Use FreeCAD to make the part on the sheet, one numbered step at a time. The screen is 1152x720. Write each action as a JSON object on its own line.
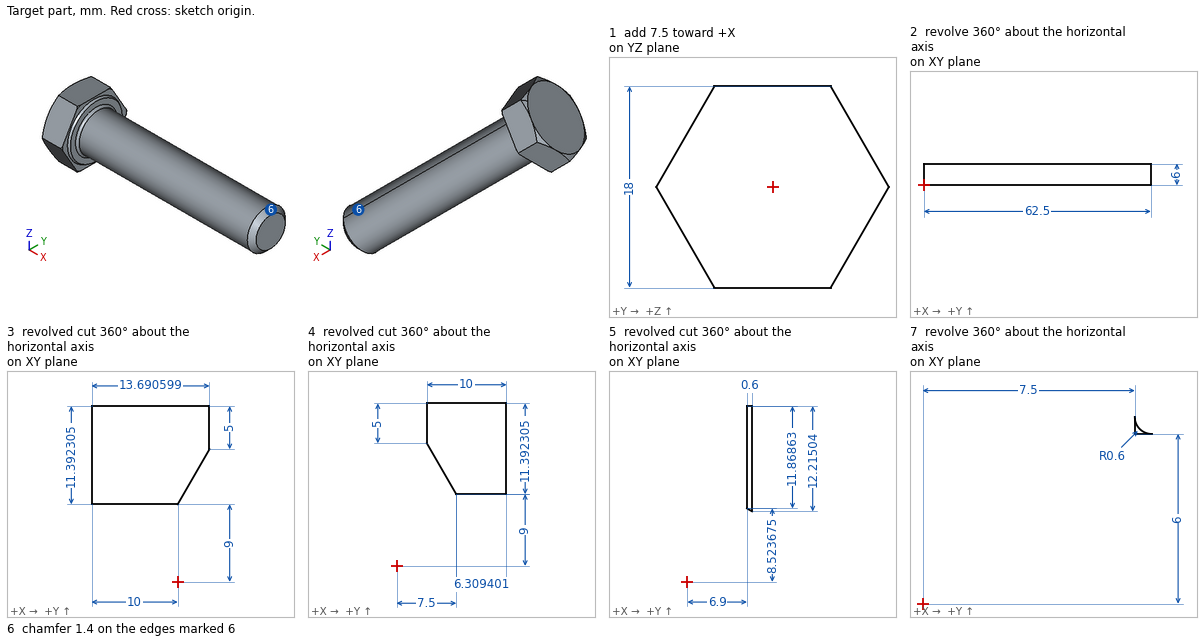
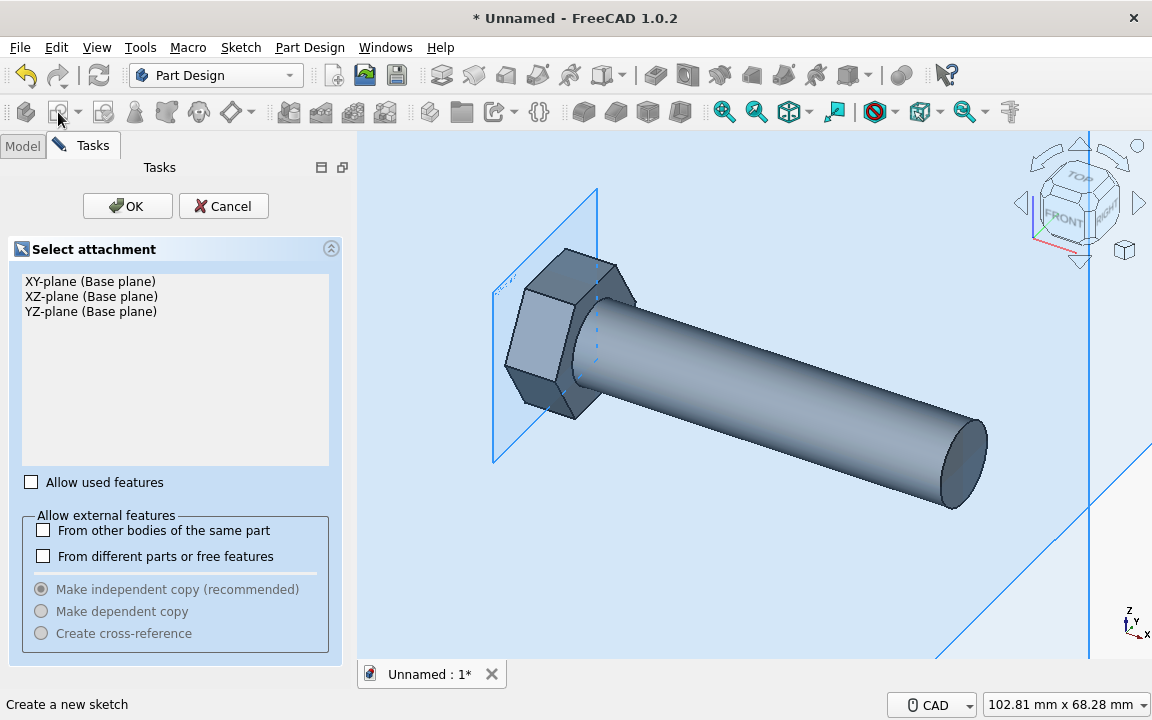
{"action": "left_click", "coordinate": [82, 282]}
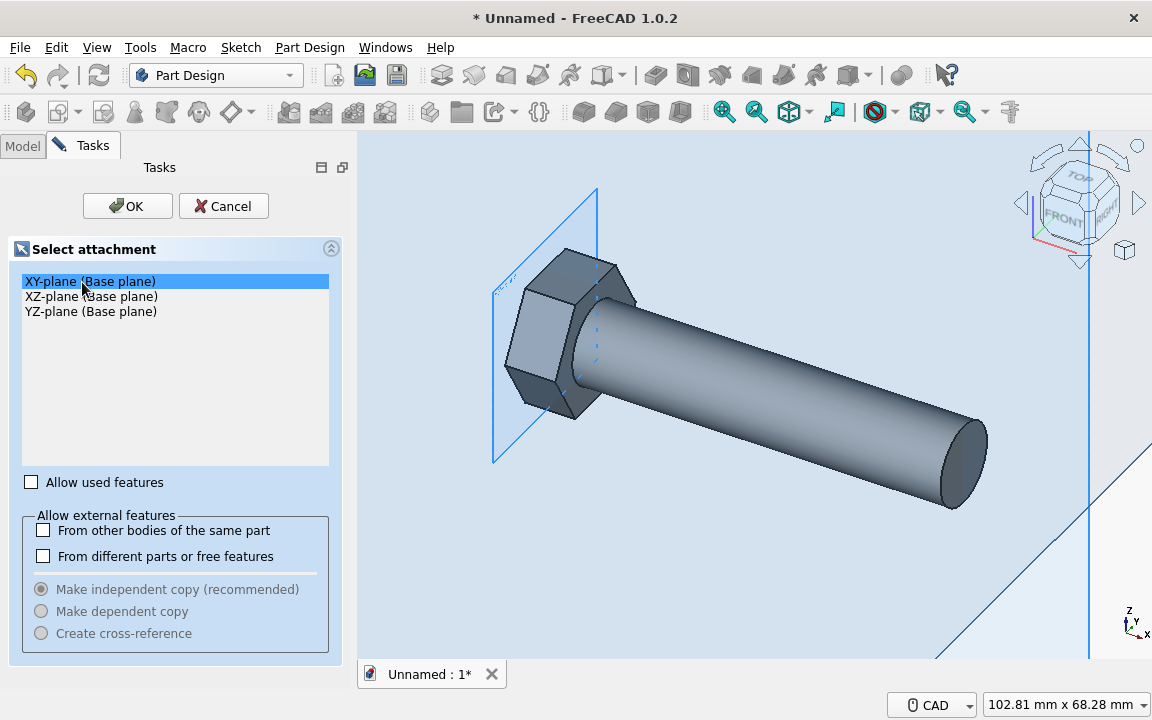
{"action": "left_click", "coordinate": [128, 206]}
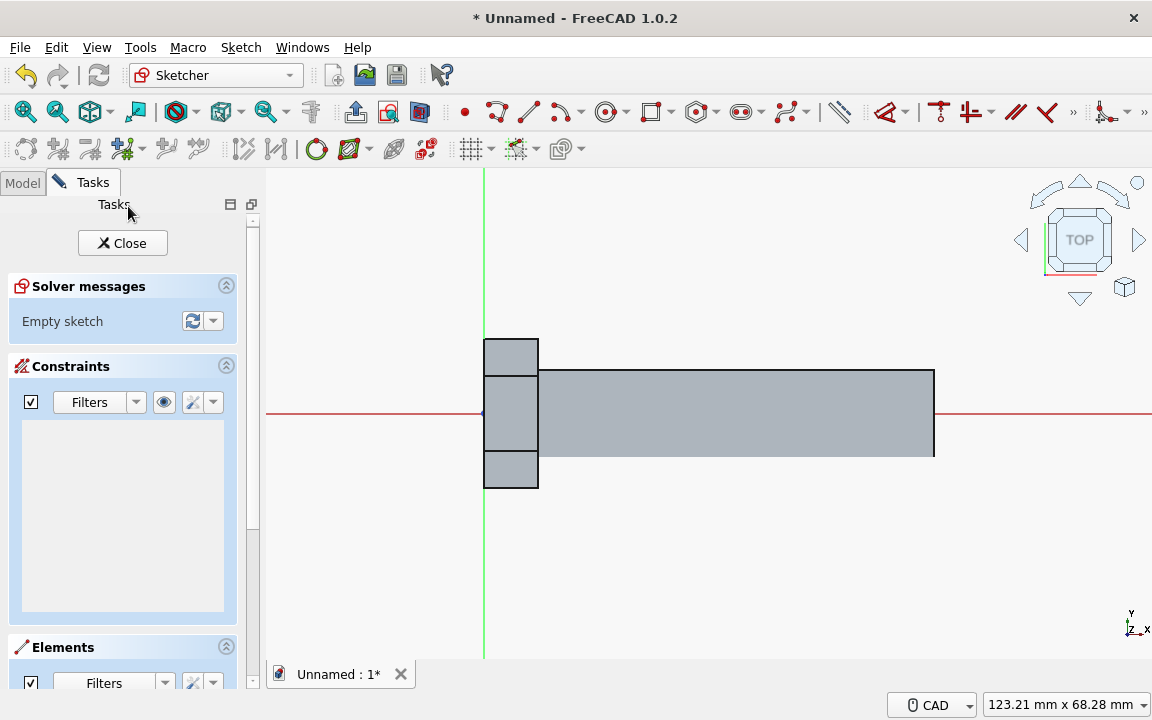
{"action": "key", "text": "q s"}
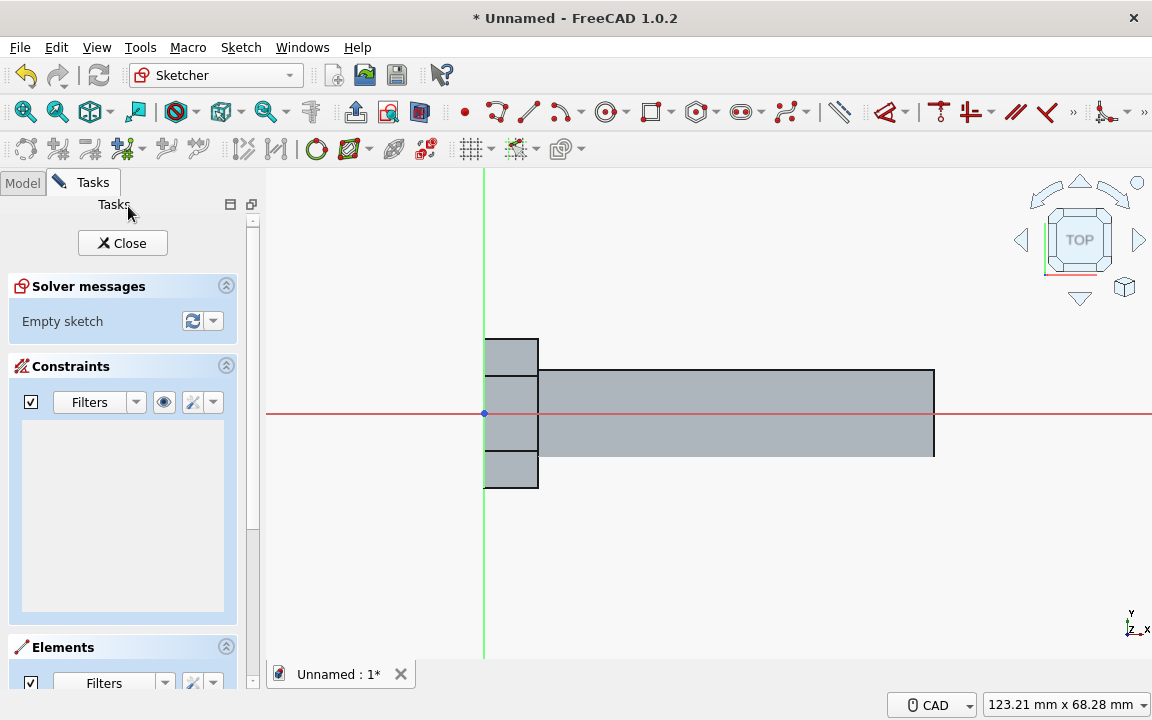
{"action": "scroll", "coordinate": [316, 280], "scroll_direction": "up", "scroll_amount": 4}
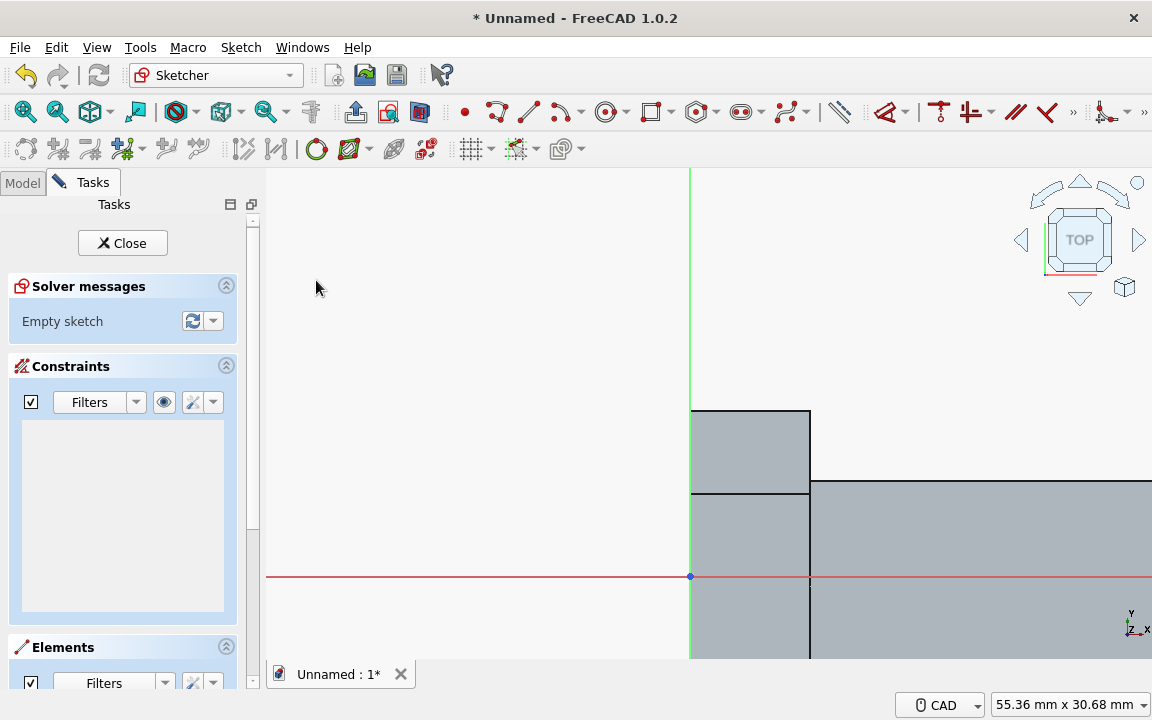
{"action": "key", "text": "g m"}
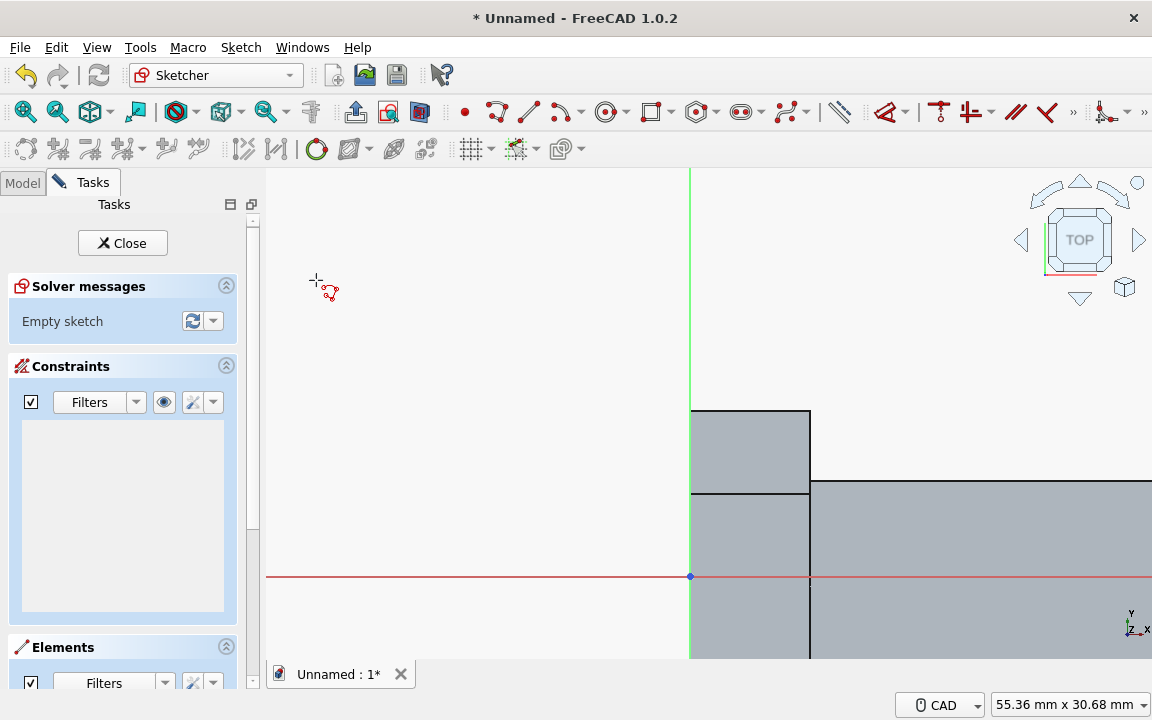
{"action": "left_click", "coordinate": [690, 433]}
{"action": "left_click", "coordinate": [750, 330]}
{"action": "left_click", "coordinate": [750, 250]}
{"action": "left_click", "coordinate": [530, 250]}
{"action": "left_click", "coordinate": [530, 433]}
{"action": "left_click", "coordinate": [690, 434]}
{"action": "key", "text": "Escape"}
{"action": "key", "text": "Escape"}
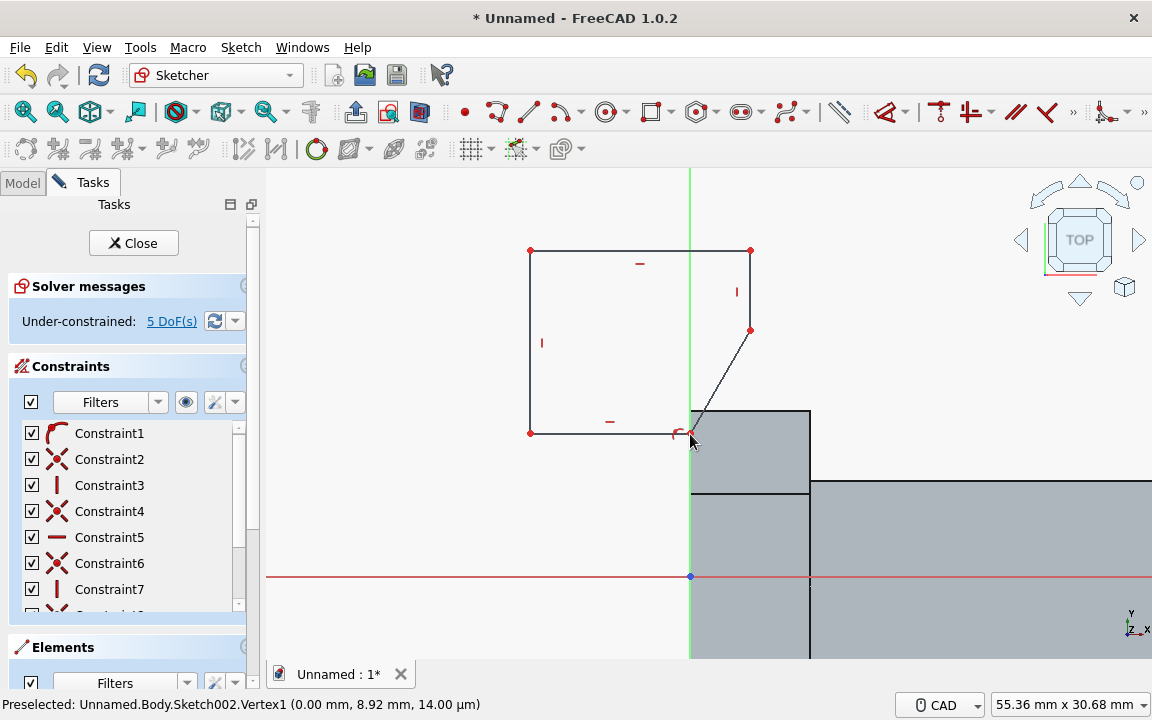
{"action": "left_click", "coordinate": [886, 112]}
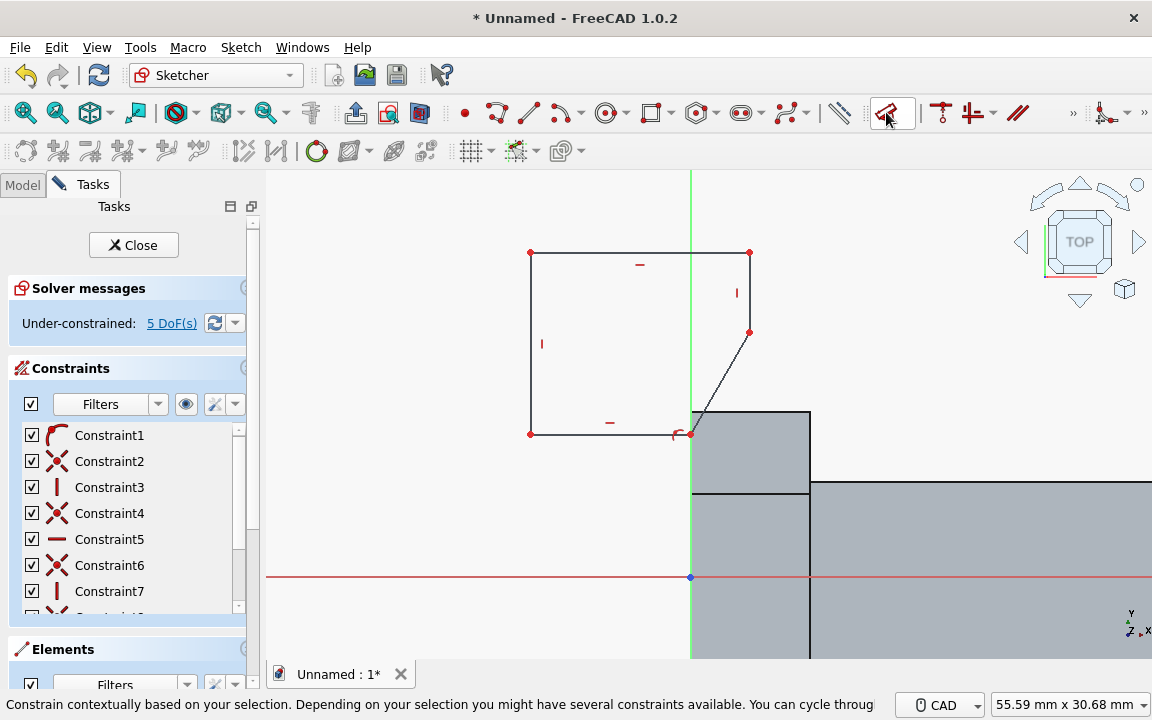
{"action": "left_click", "coordinate": [750, 308]}
{"action": "left_click", "coordinate": [784, 292]}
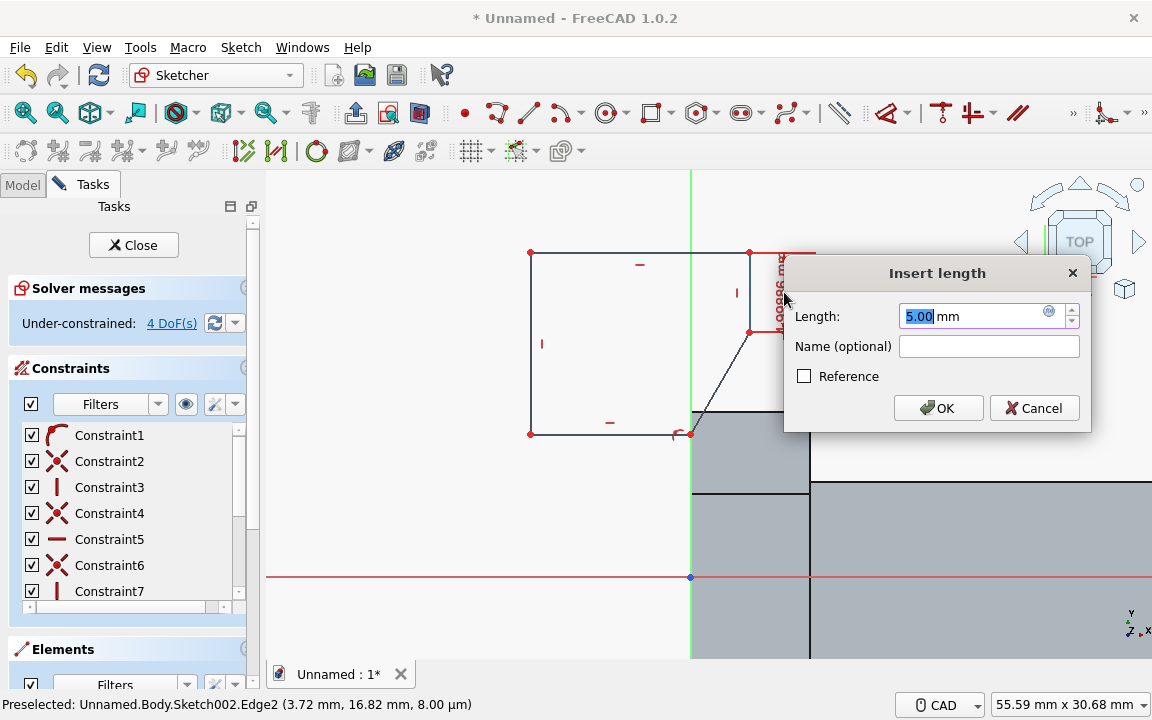
{"action": "type", "text": "5"}
{"action": "key", "text": "Return"}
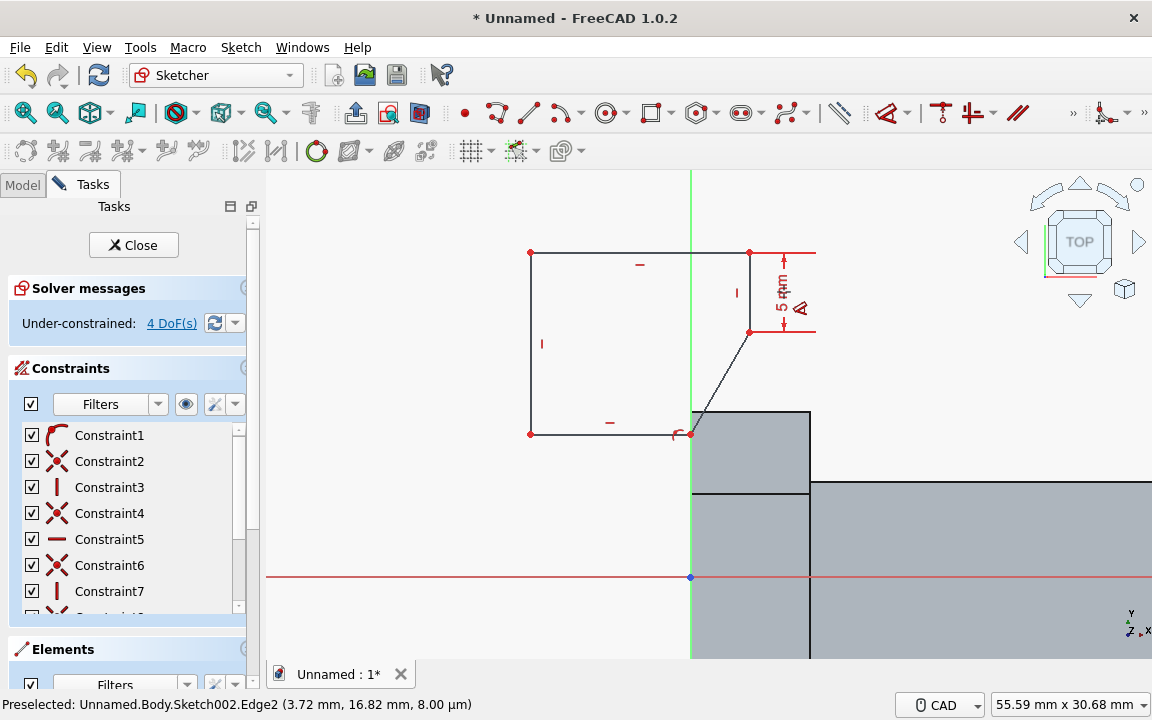
{"action": "left_click", "coordinate": [579, 435]}
{"action": "left_click", "coordinate": [611, 469]}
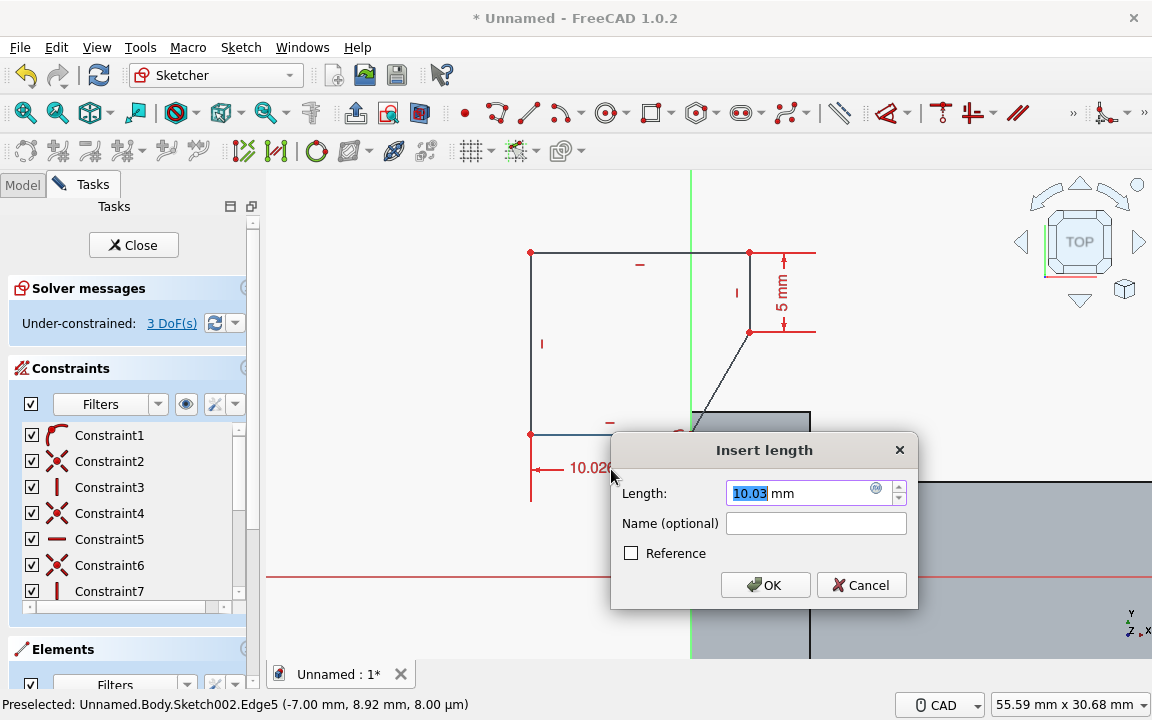
{"action": "type", "text": "10"}
{"action": "key", "text": "Return"}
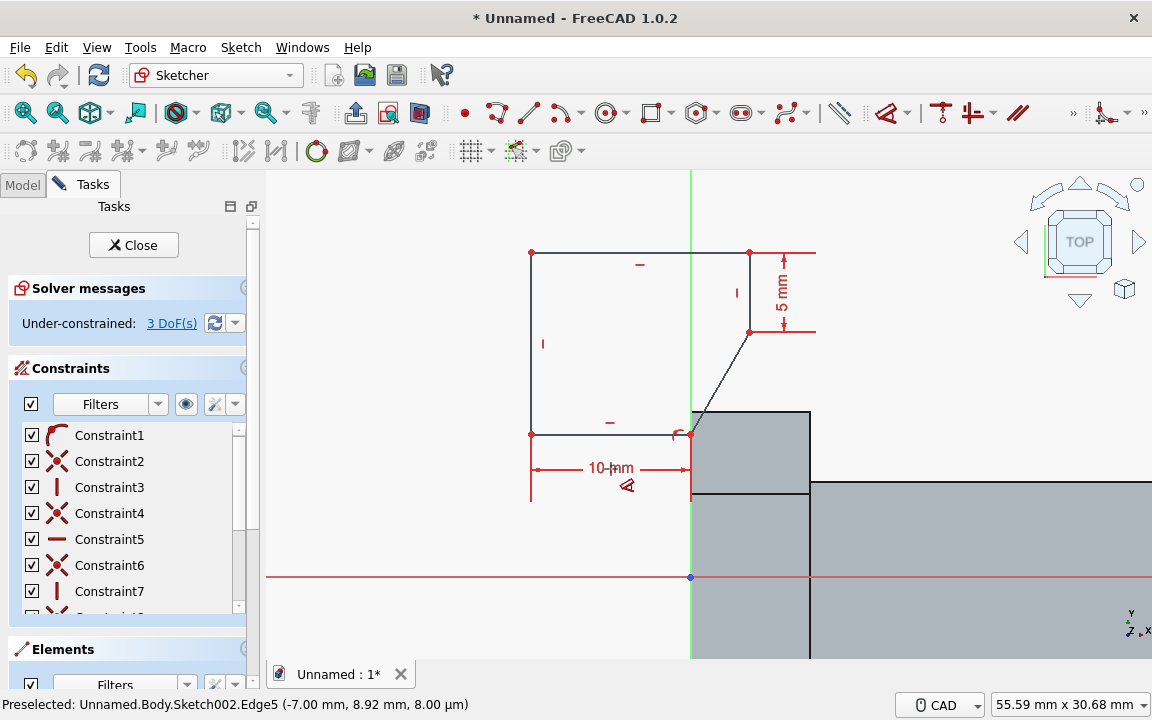
{"action": "left_click", "coordinate": [691, 435]}
{"action": "left_click", "coordinate": [725, 506]}